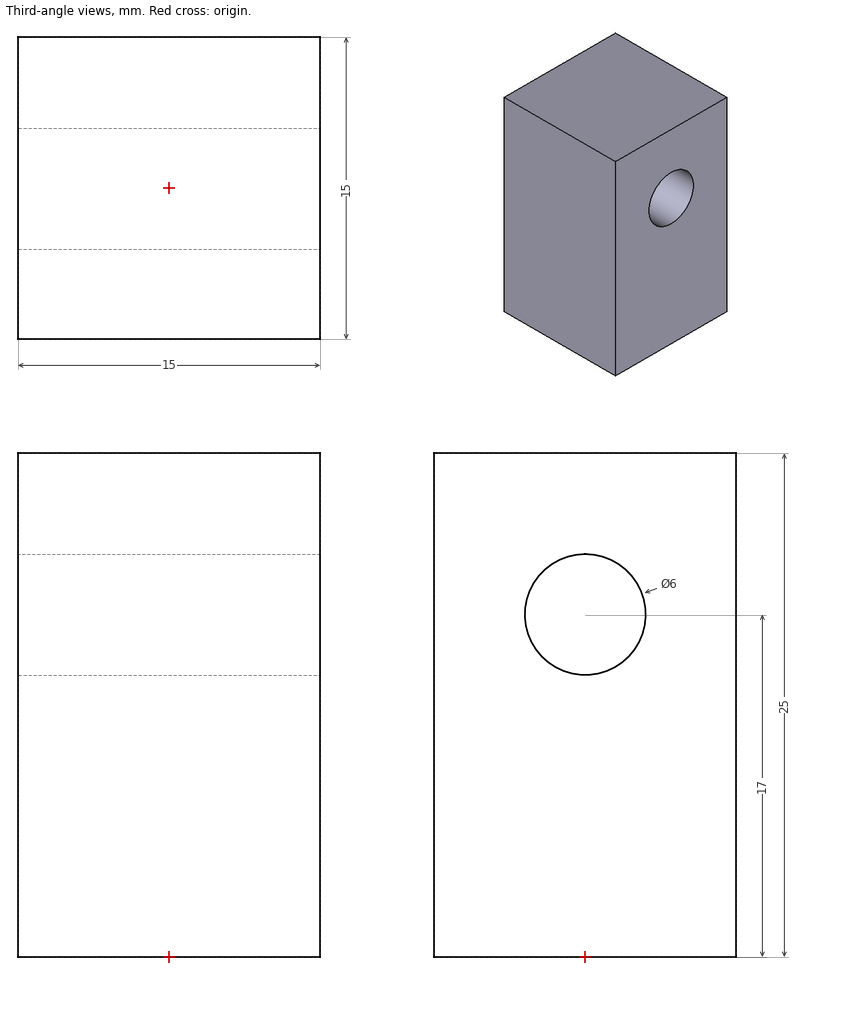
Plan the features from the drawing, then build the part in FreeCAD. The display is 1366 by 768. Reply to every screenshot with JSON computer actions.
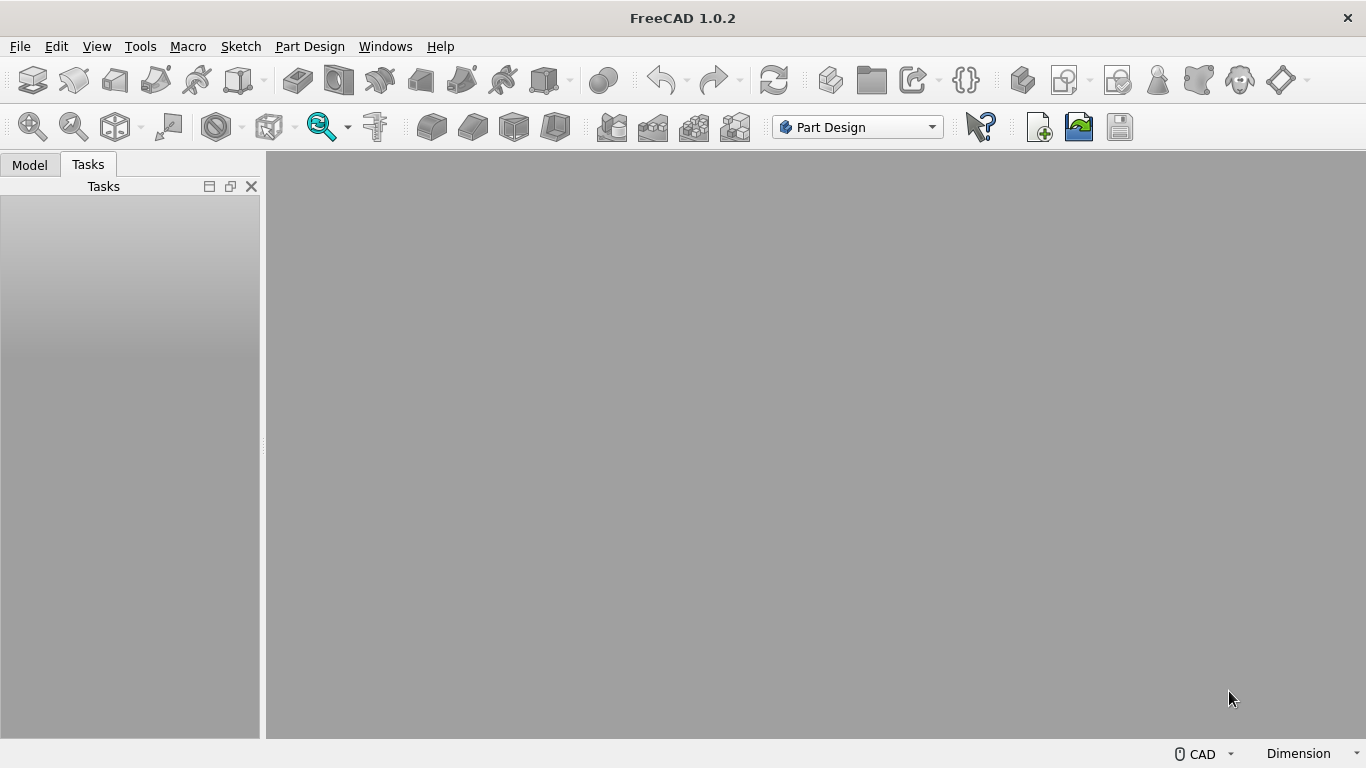
{"action": "left_click", "coordinate": [1038, 128]}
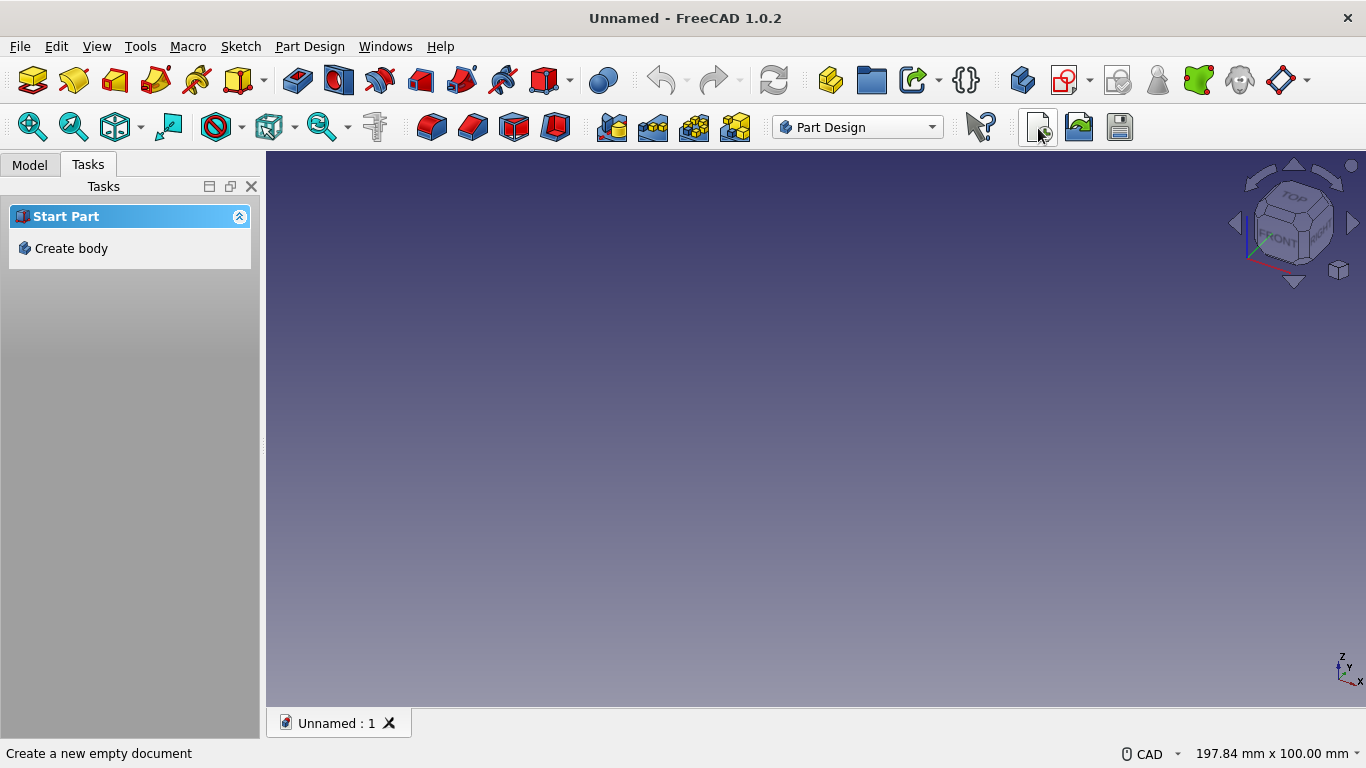
{"action": "left_click", "coordinate": [1064, 80]}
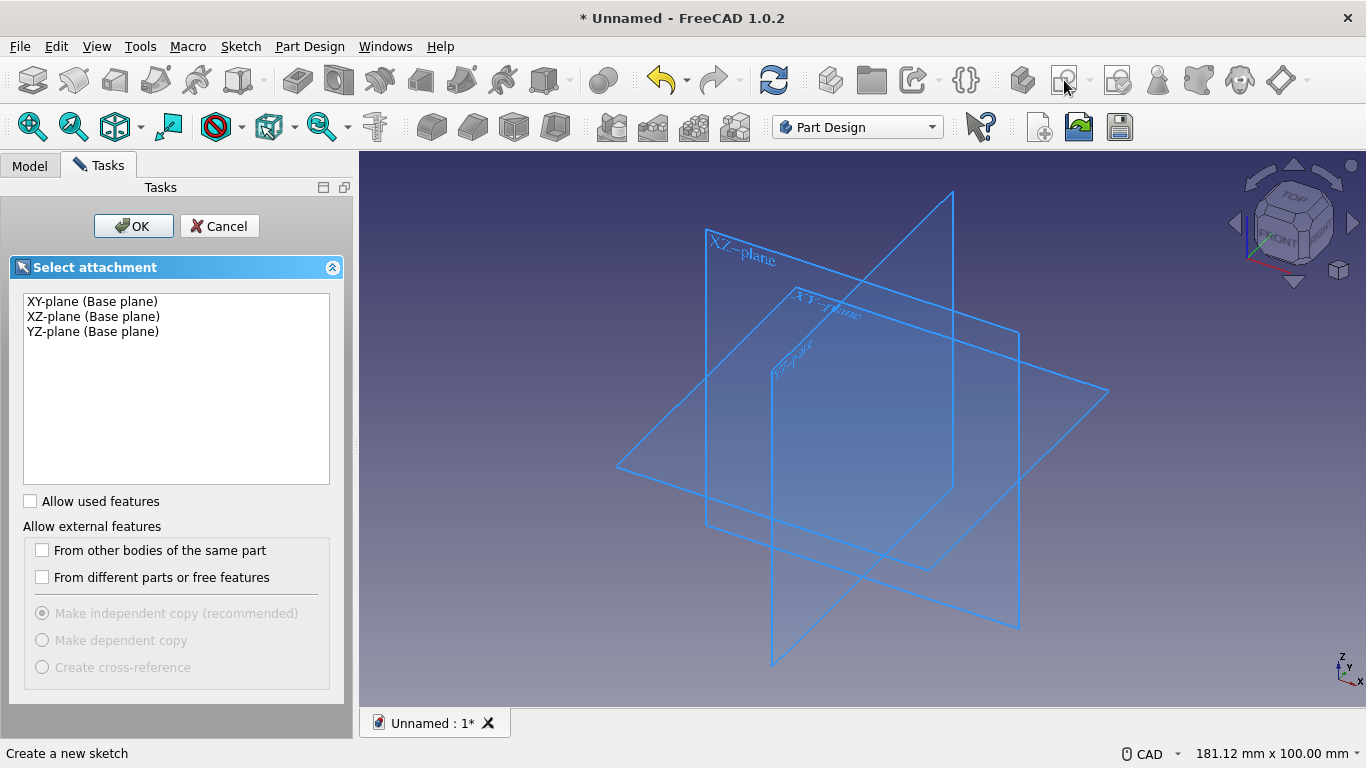
{"action": "left_click", "coordinate": [84, 302]}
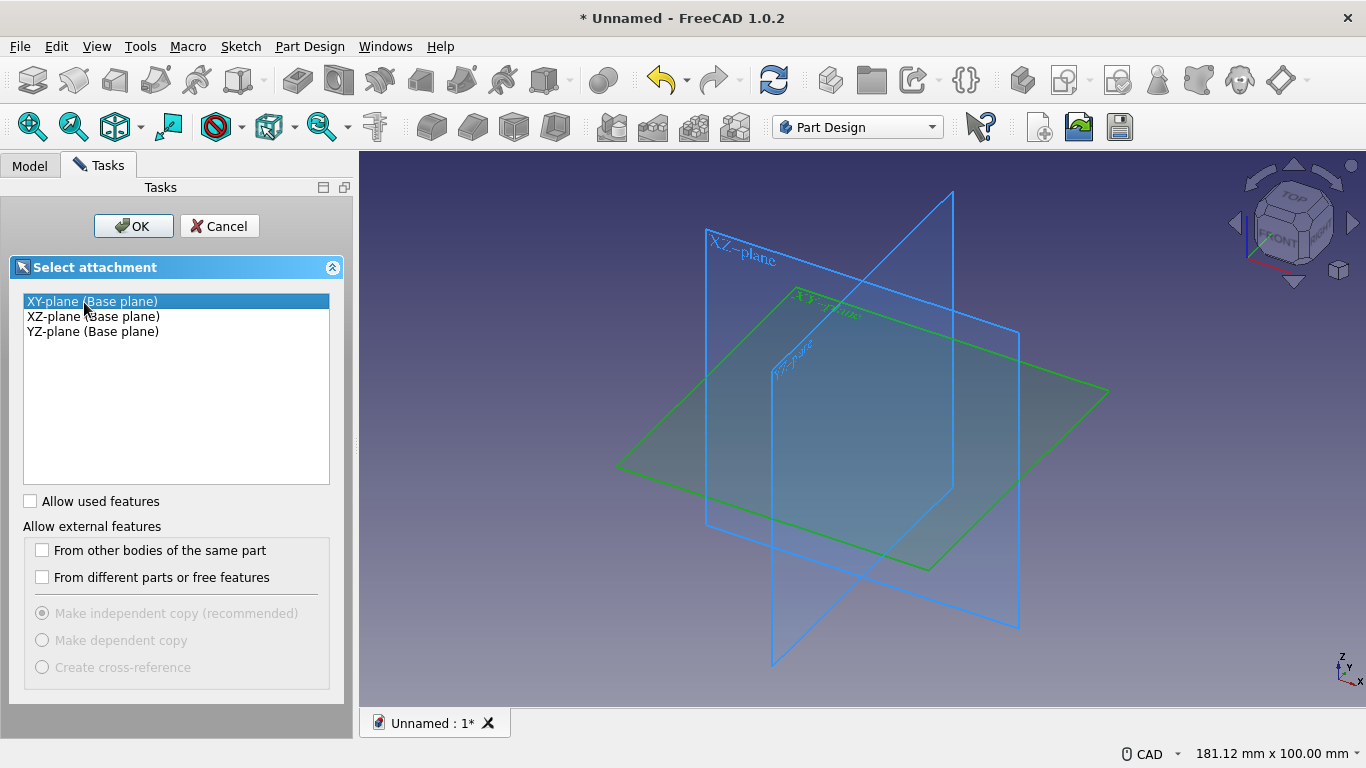
{"action": "left_click", "coordinate": [134, 226]}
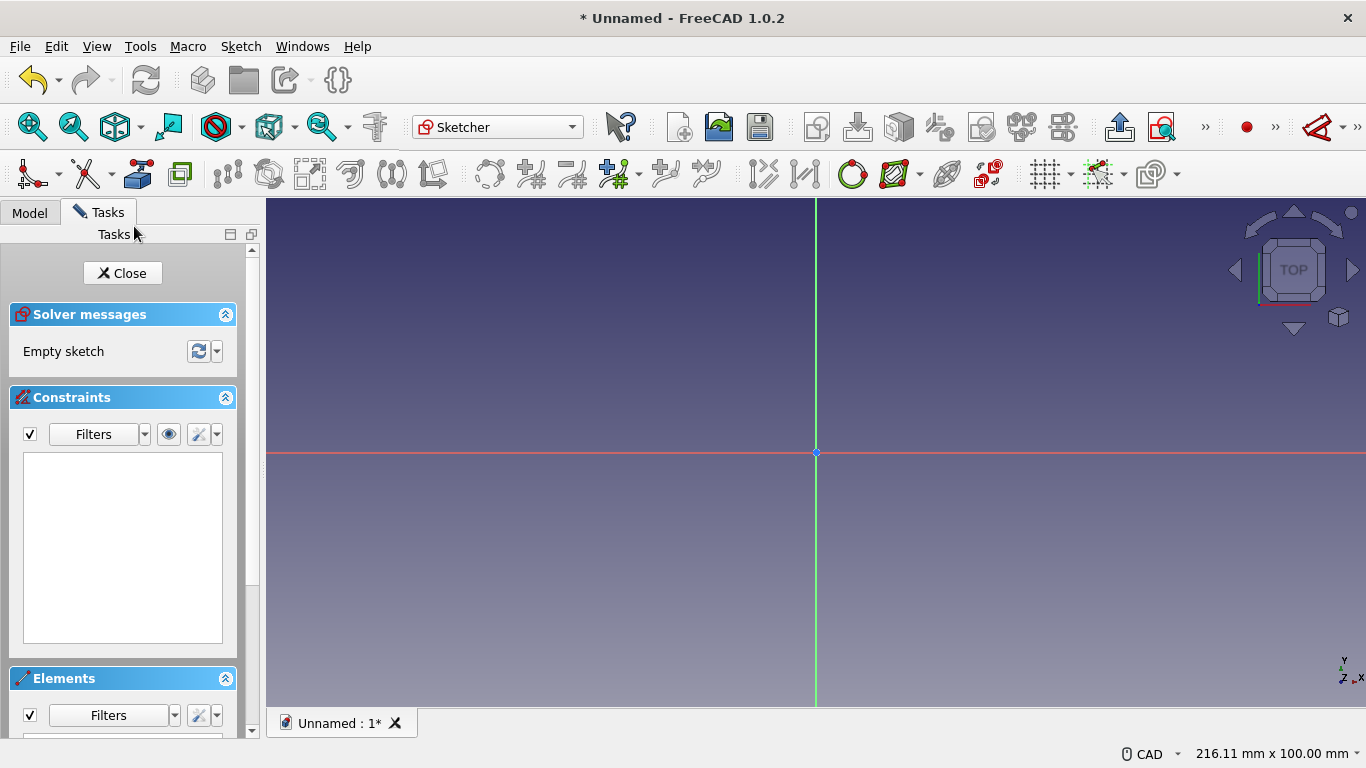
{"action": "scroll", "coordinate": [838, 452], "scroll_direction": "up", "scroll_amount": 7}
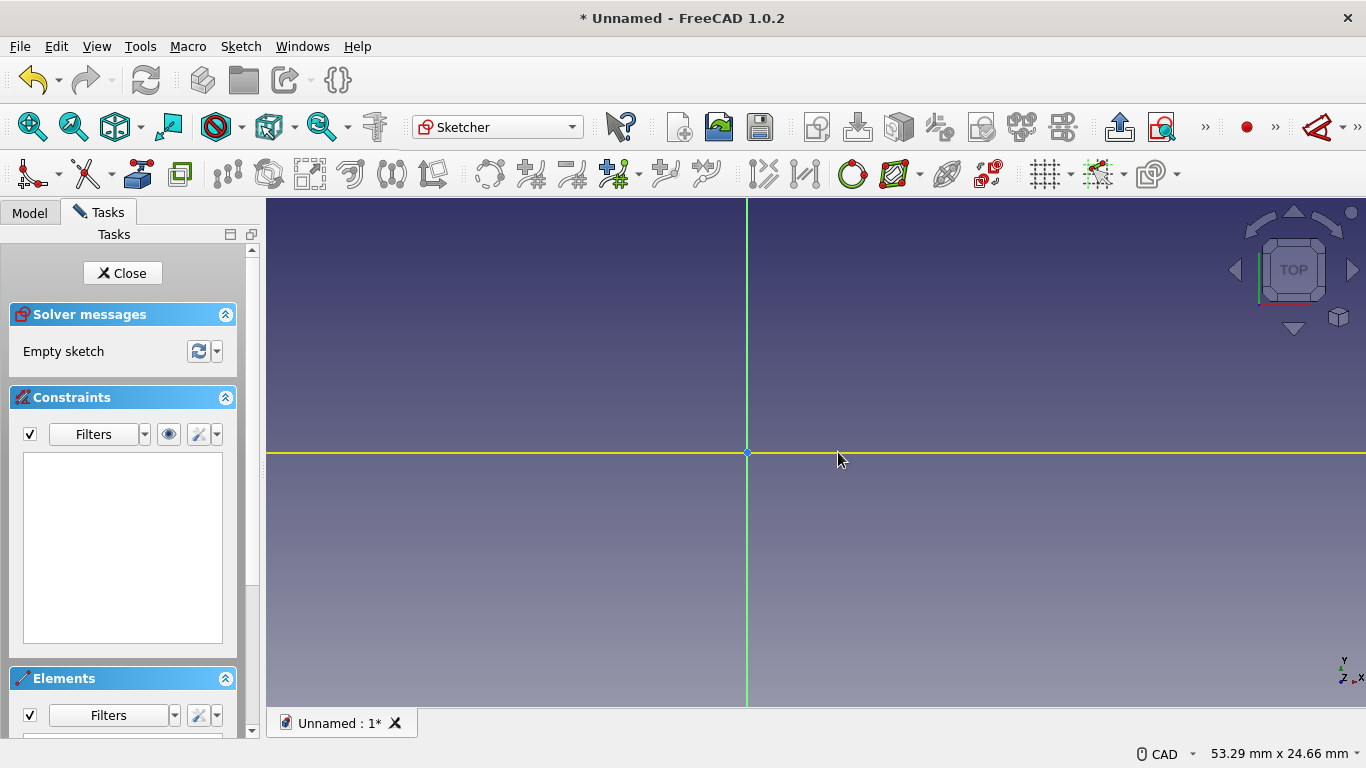
{"action": "key", "text": "g v"}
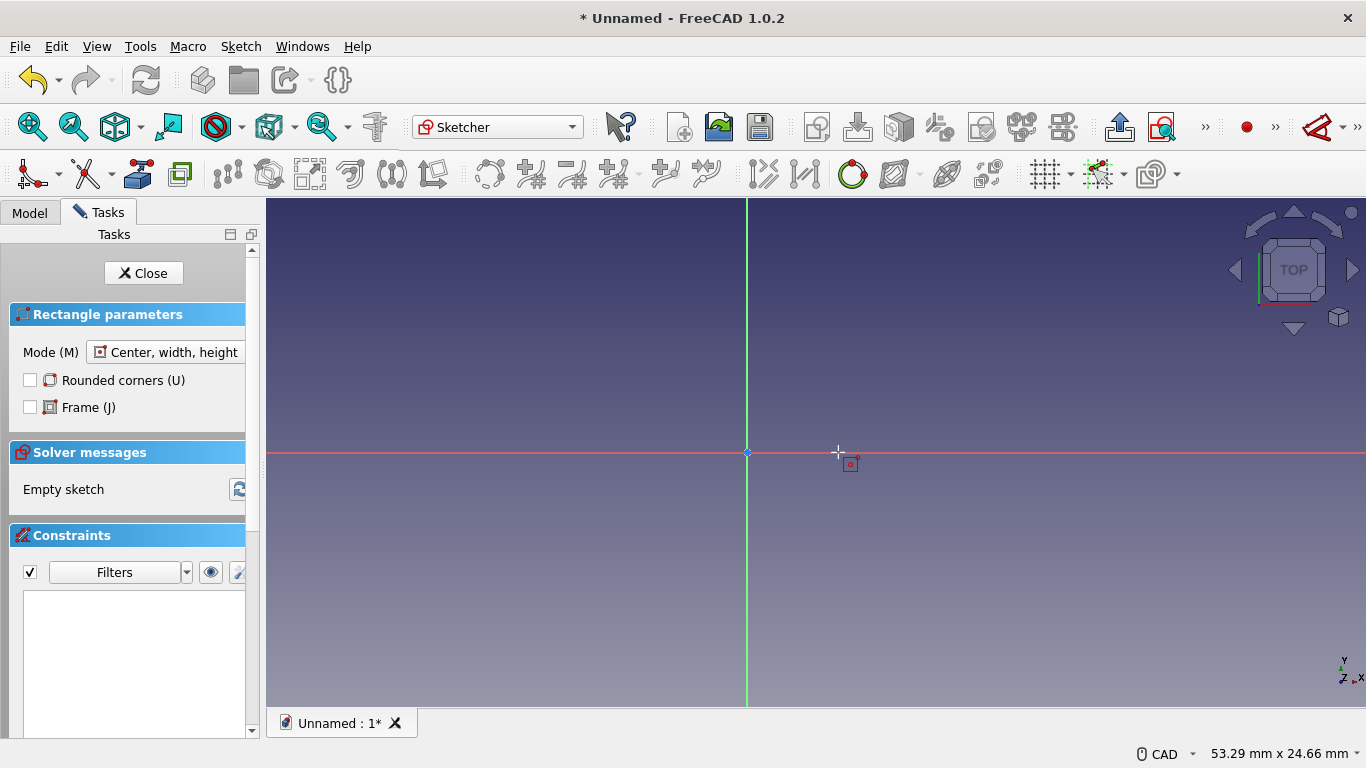
{"action": "left_click", "coordinate": [747, 452]}
{"action": "mouse_move", "coordinate": [902, 298]}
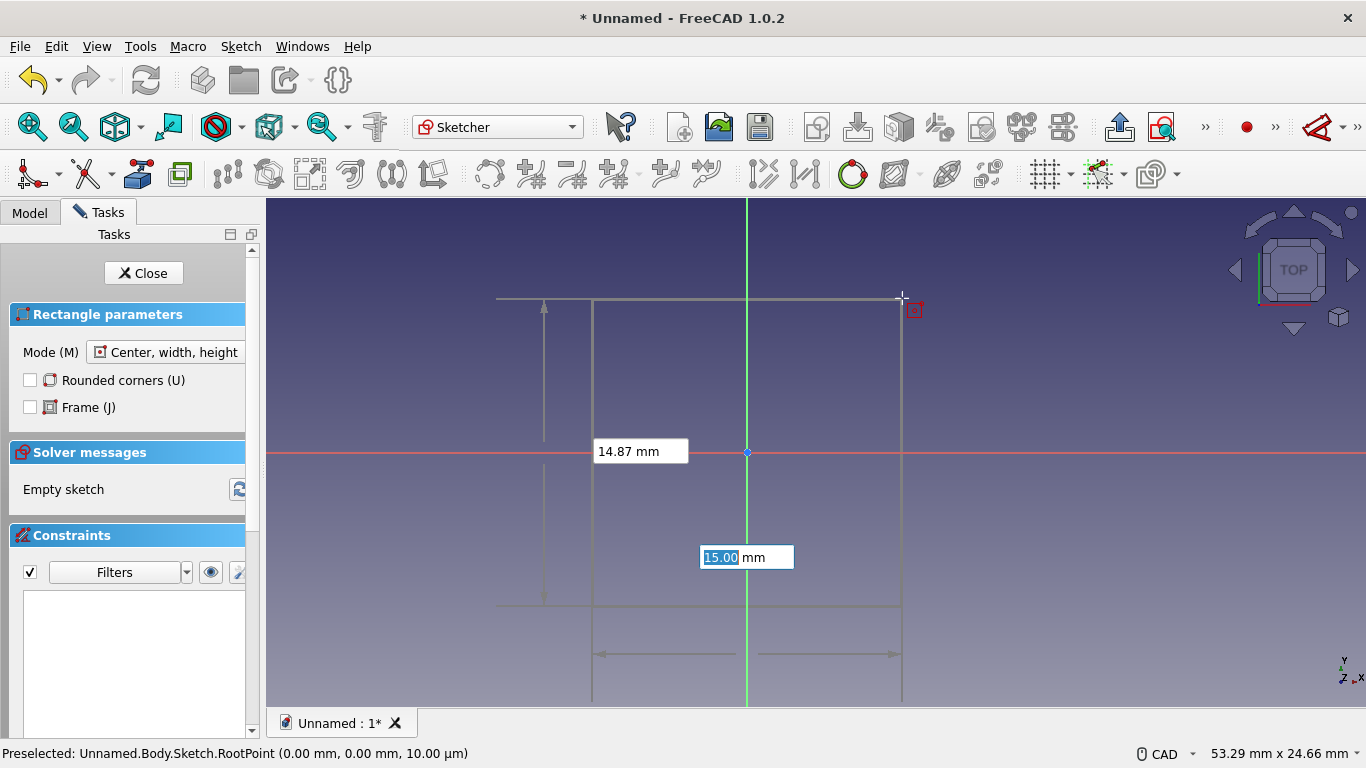
{"action": "type", "text": "15"}
{"action": "key", "text": "Tab"}
{"action": "type", "text": "15"}
{"action": "key", "text": "Return"}
{"action": "key", "text": "Escape"}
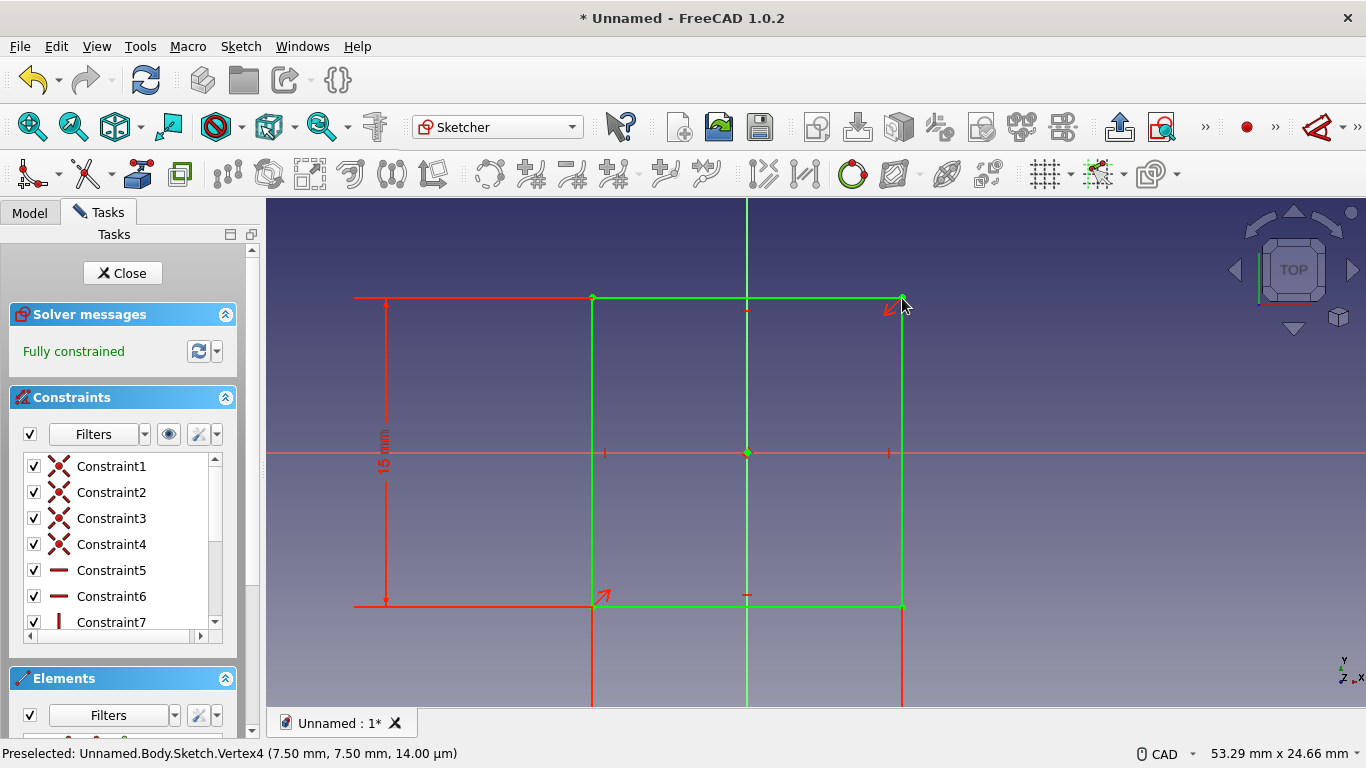
{"action": "left_click", "coordinate": [123, 273]}